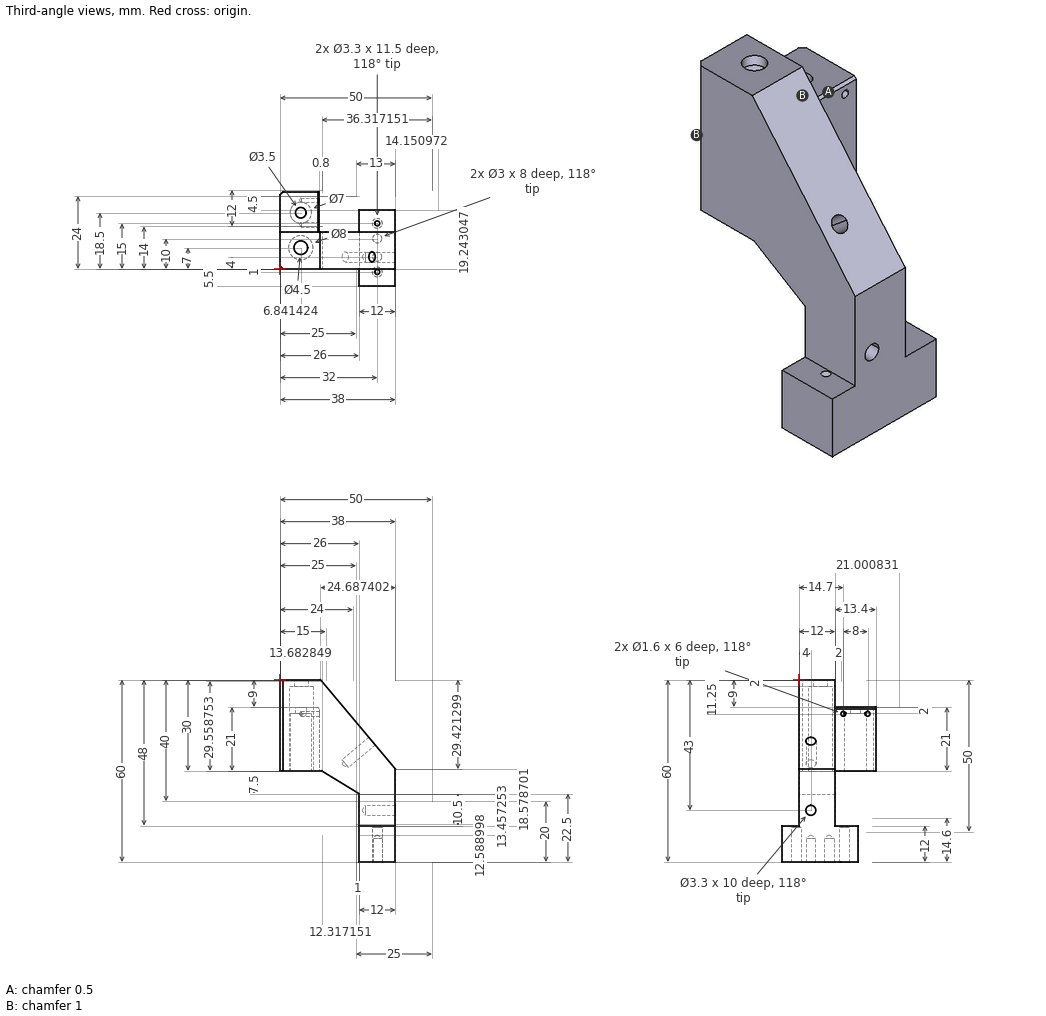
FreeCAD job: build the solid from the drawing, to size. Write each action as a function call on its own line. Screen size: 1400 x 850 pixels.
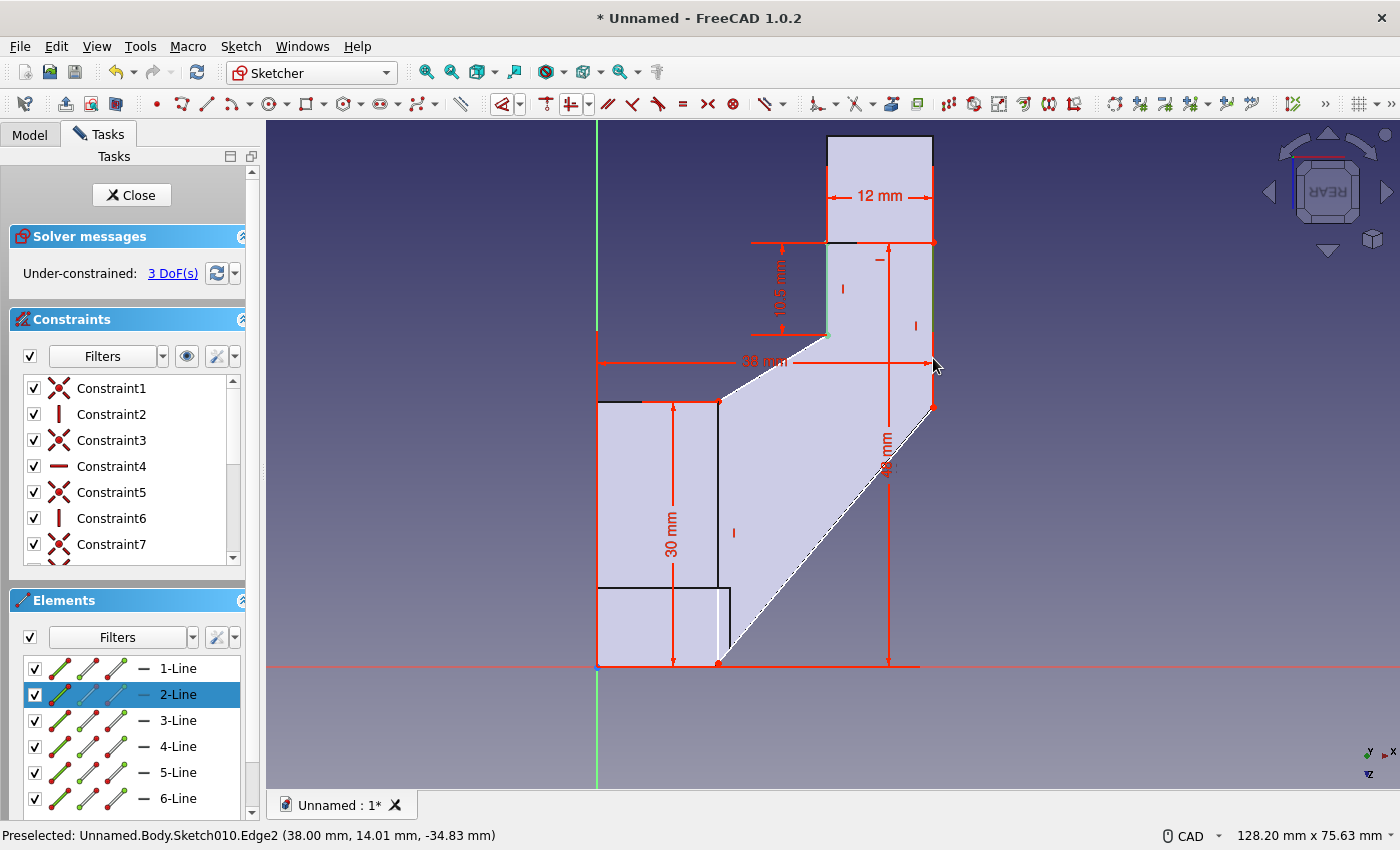
key(i)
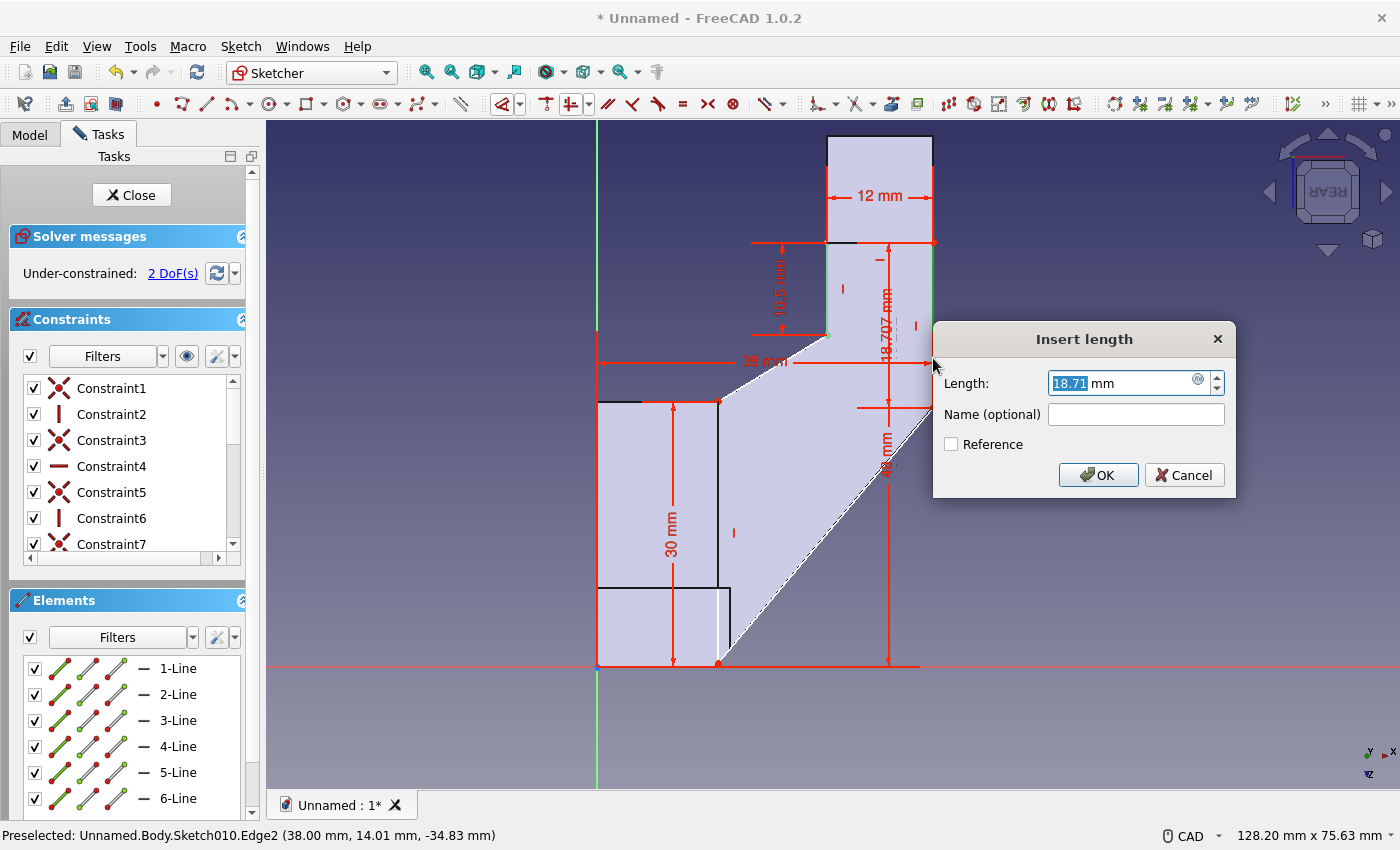
text(18.578701)
key(Return)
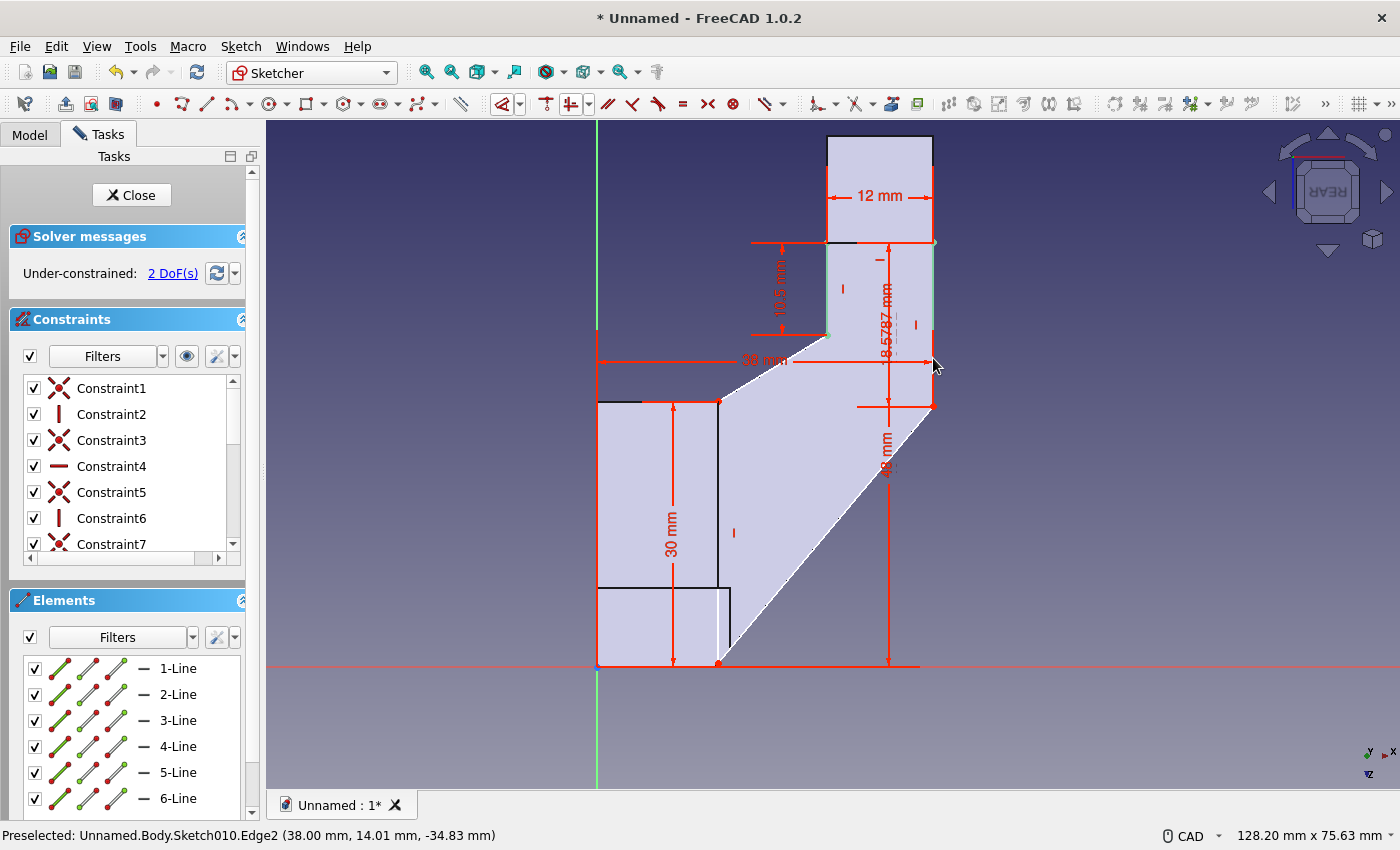
click(718, 480)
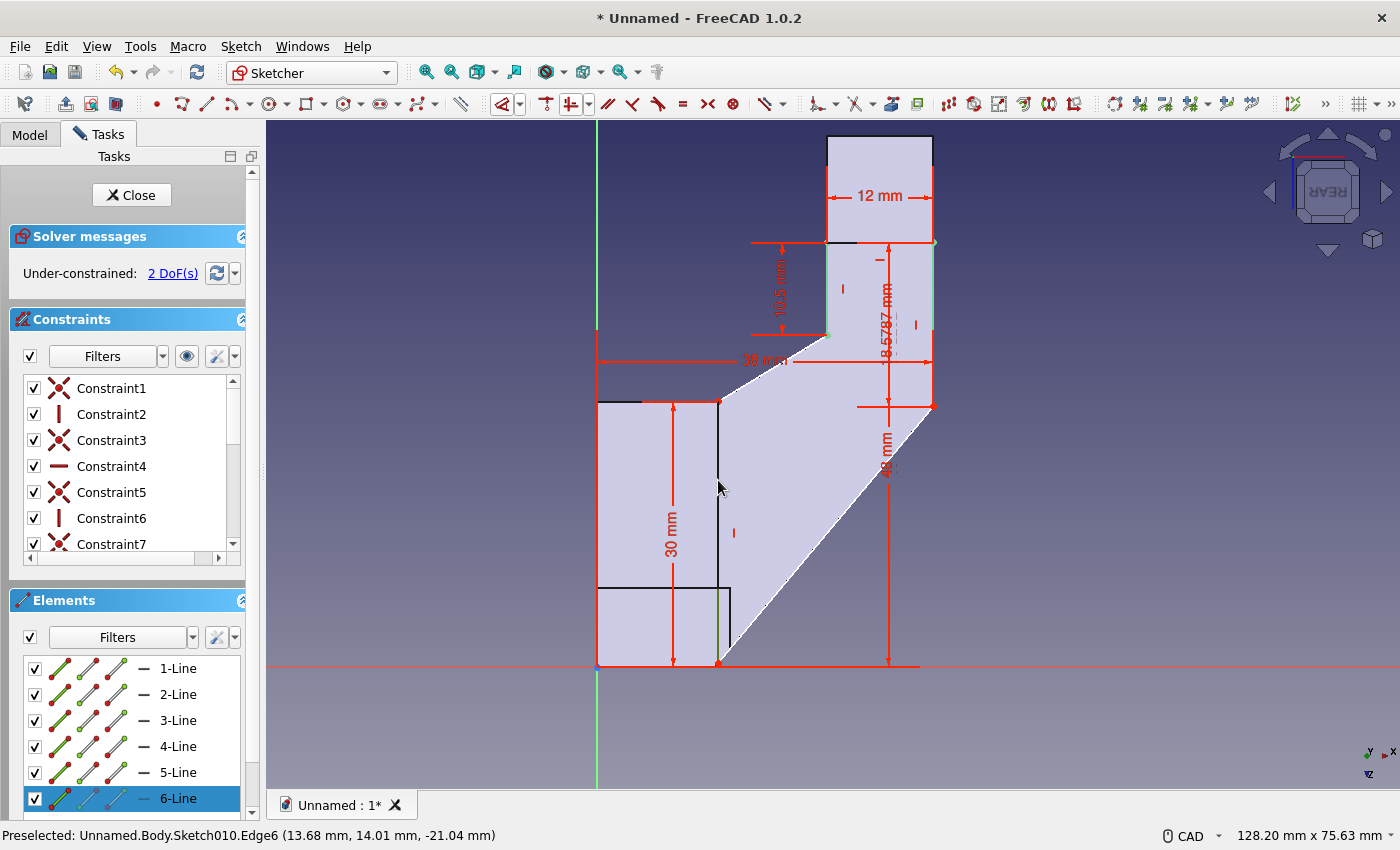
click(520, 104)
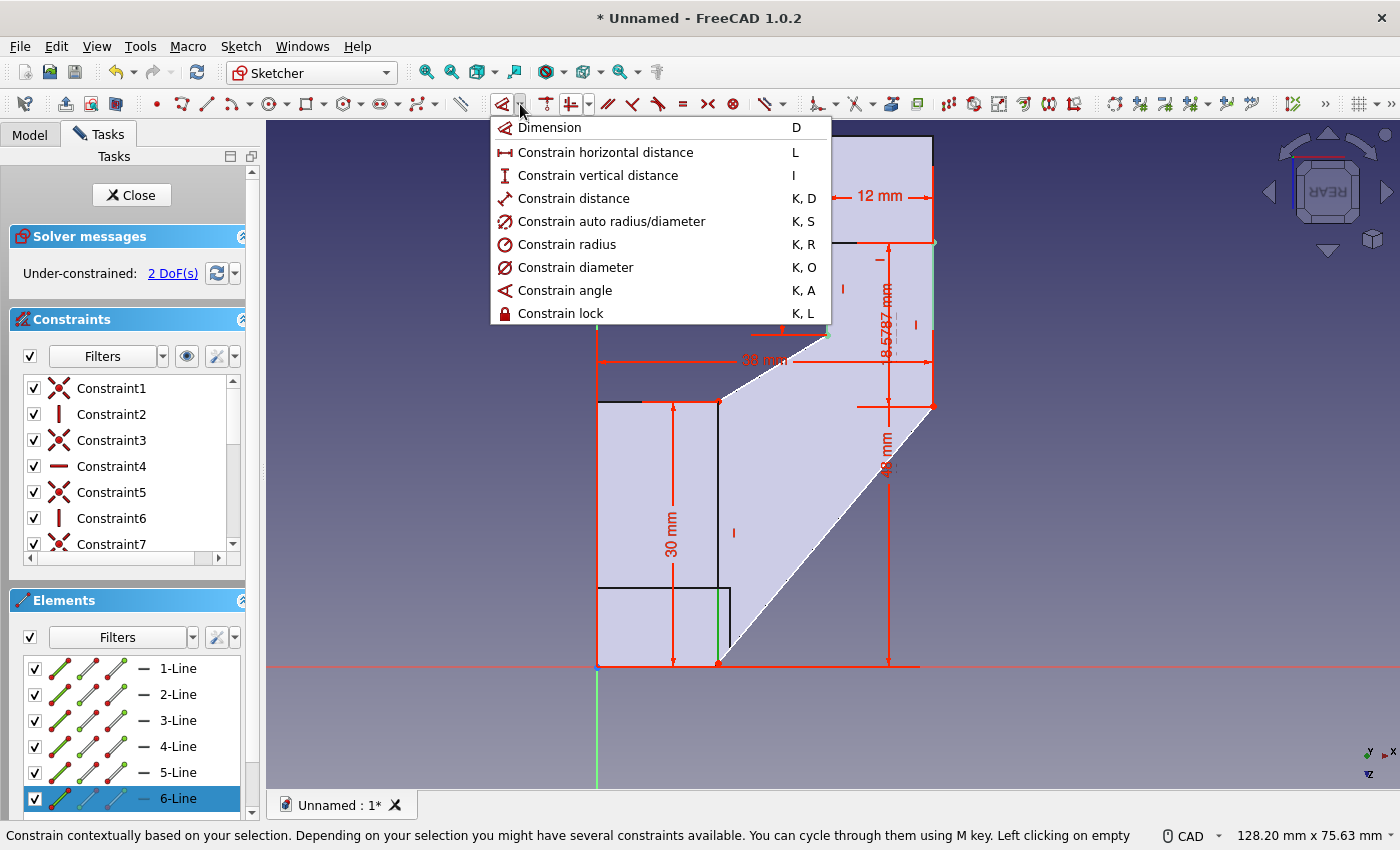
click(661, 176)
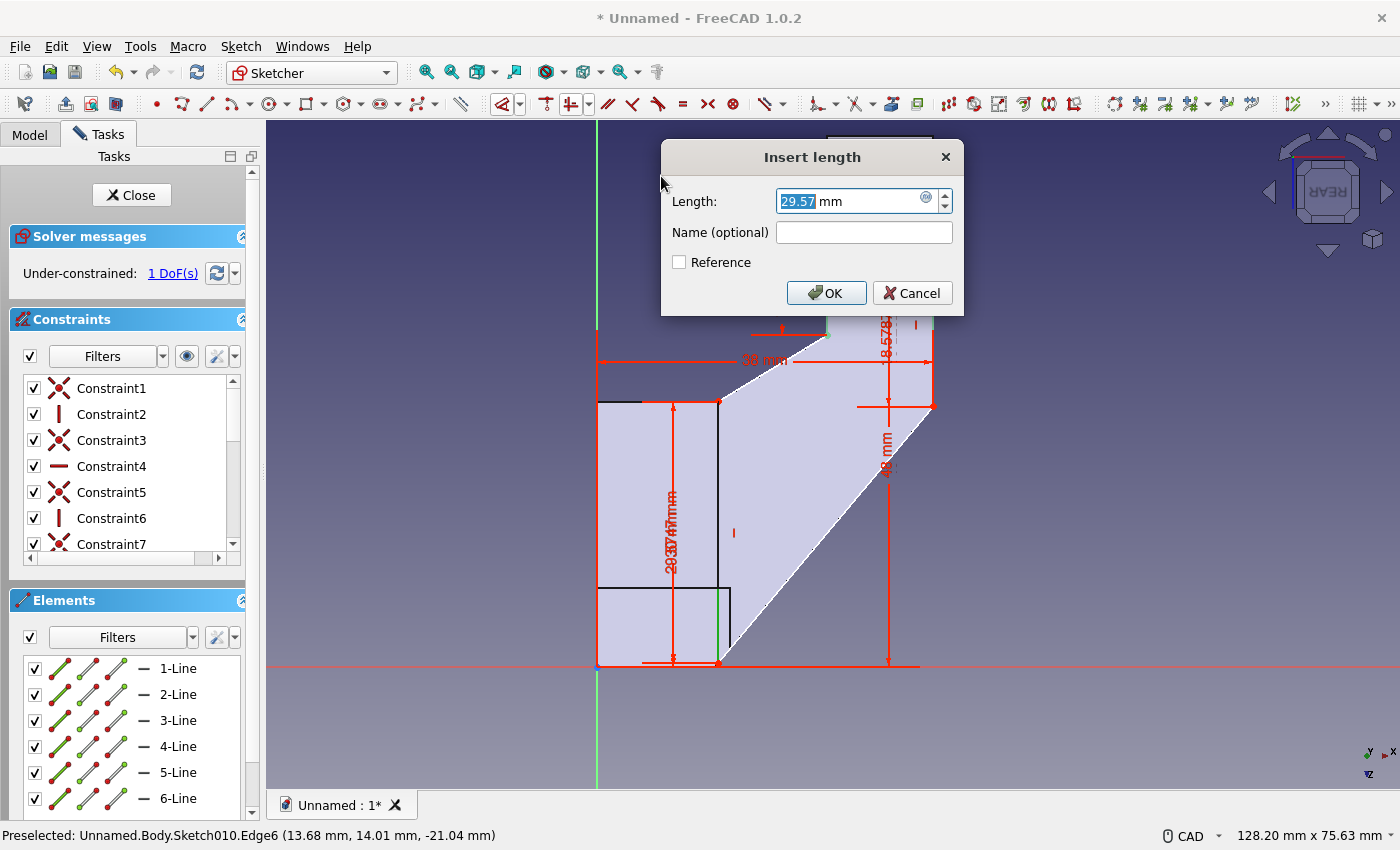
text(29.558753)
key(Return)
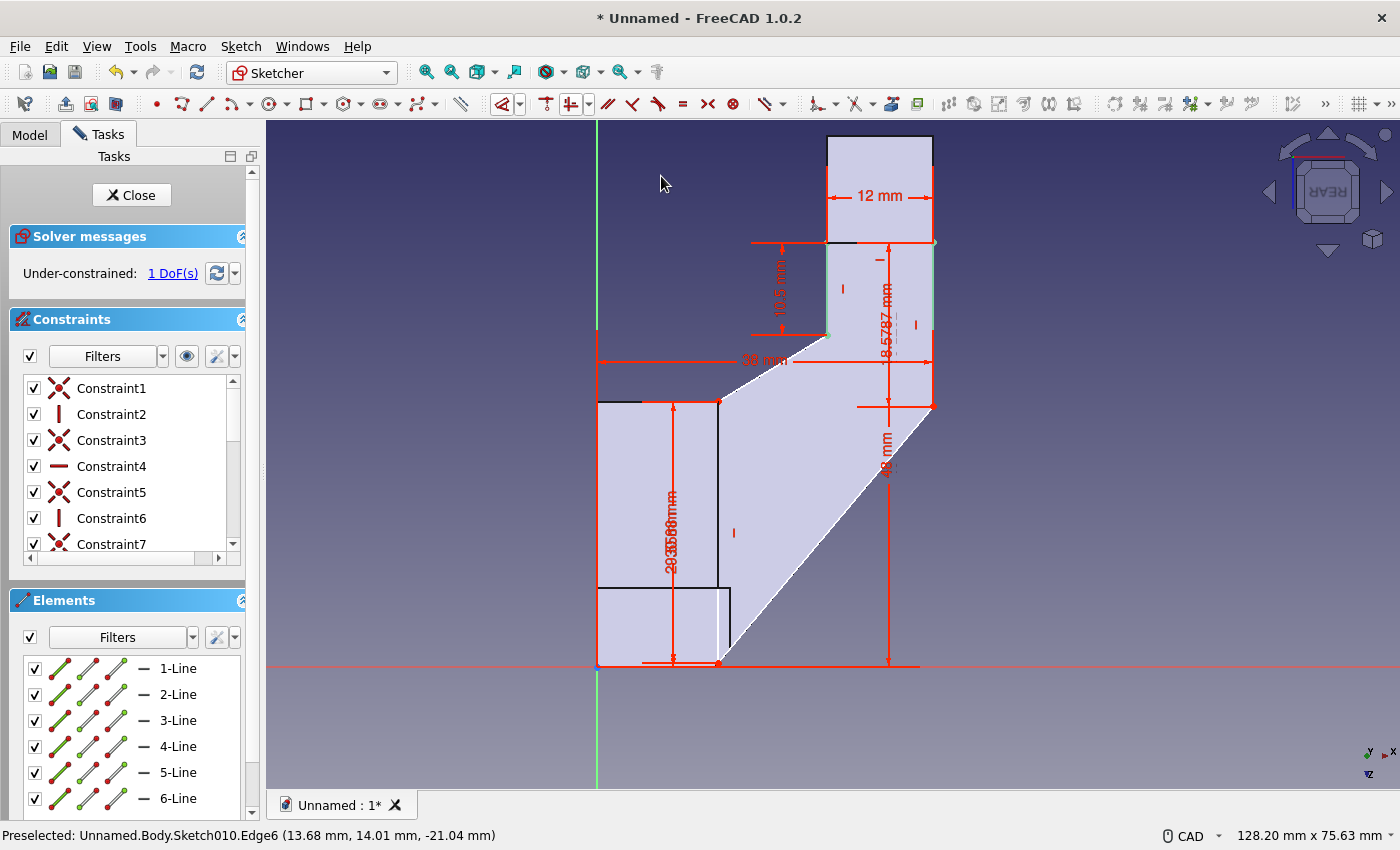
click(718, 663)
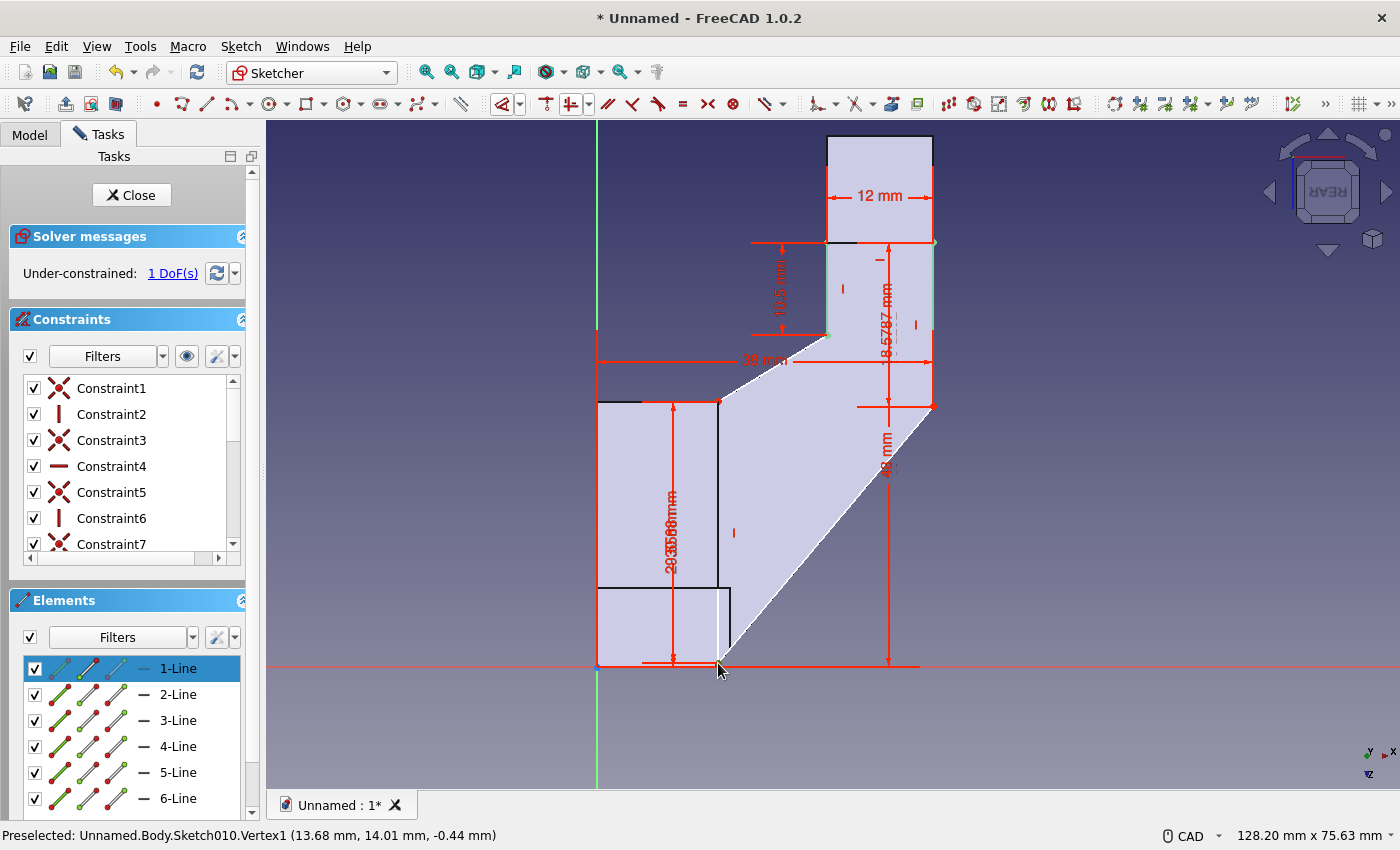
key(l)